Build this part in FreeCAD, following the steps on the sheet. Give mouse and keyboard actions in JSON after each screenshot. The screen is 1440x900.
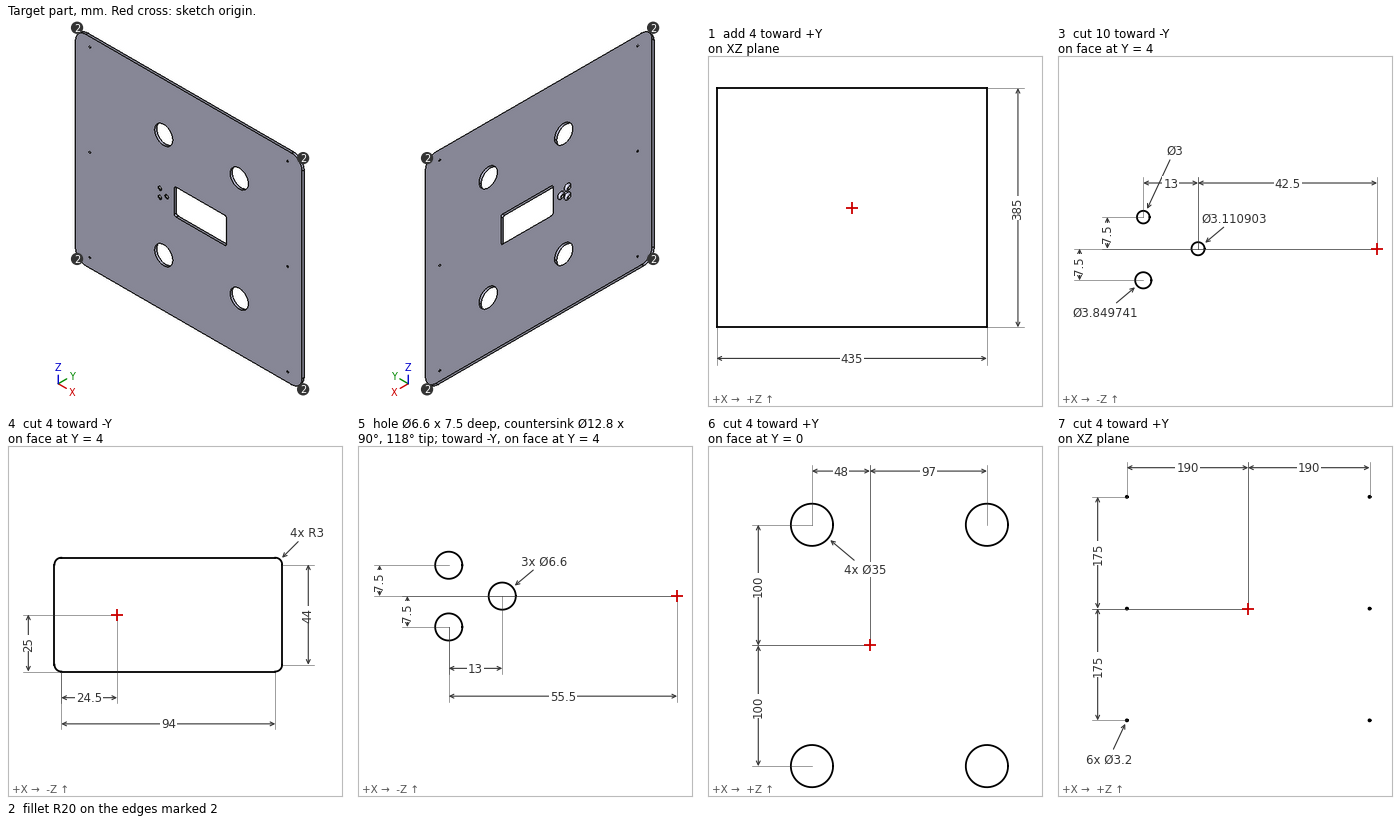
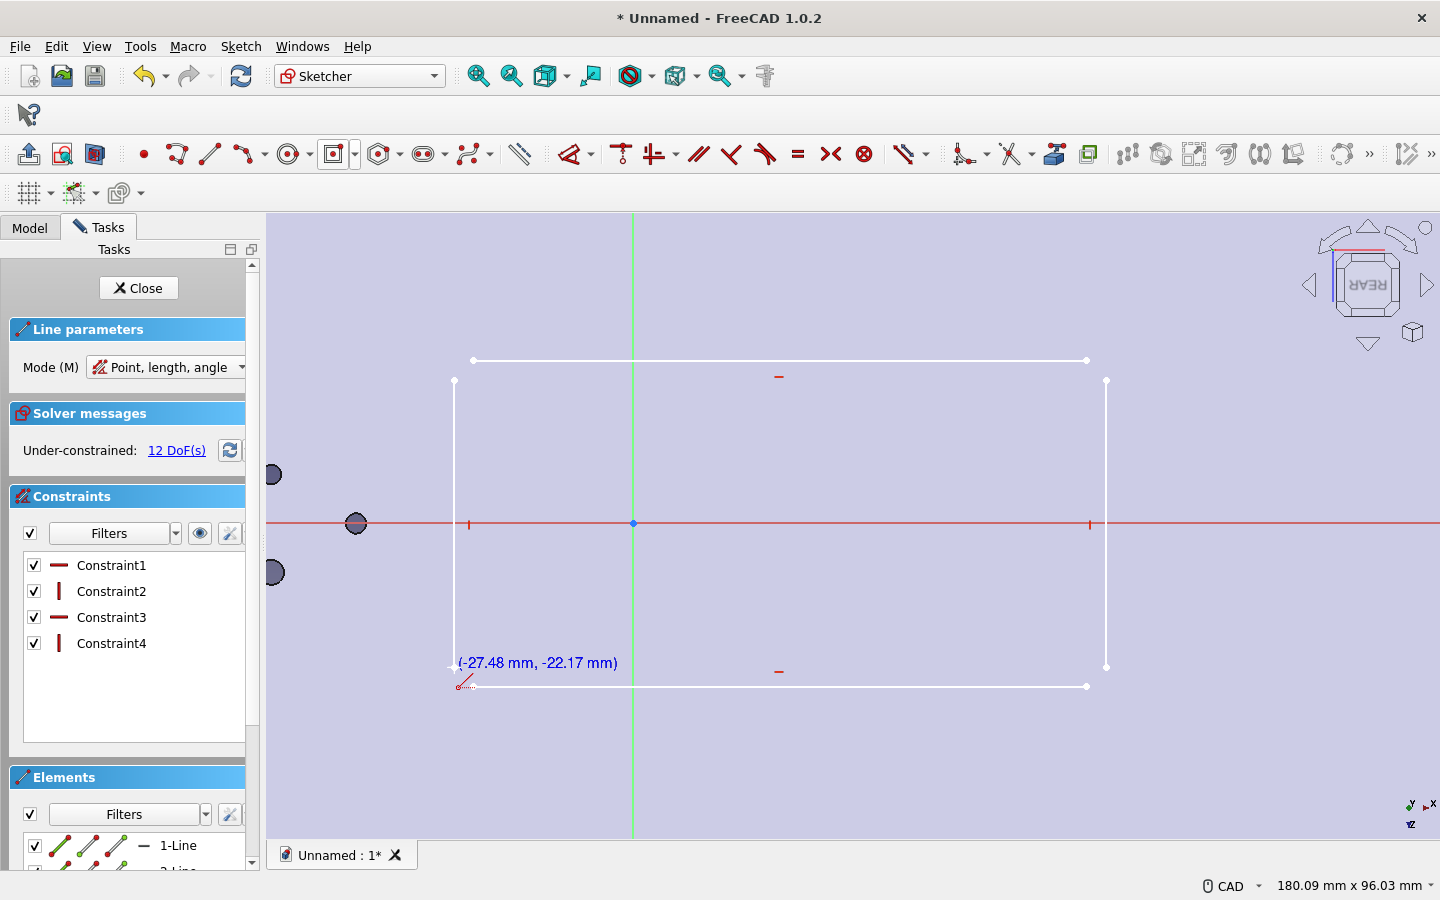
{"action": "left_click", "coordinate": [242, 154]}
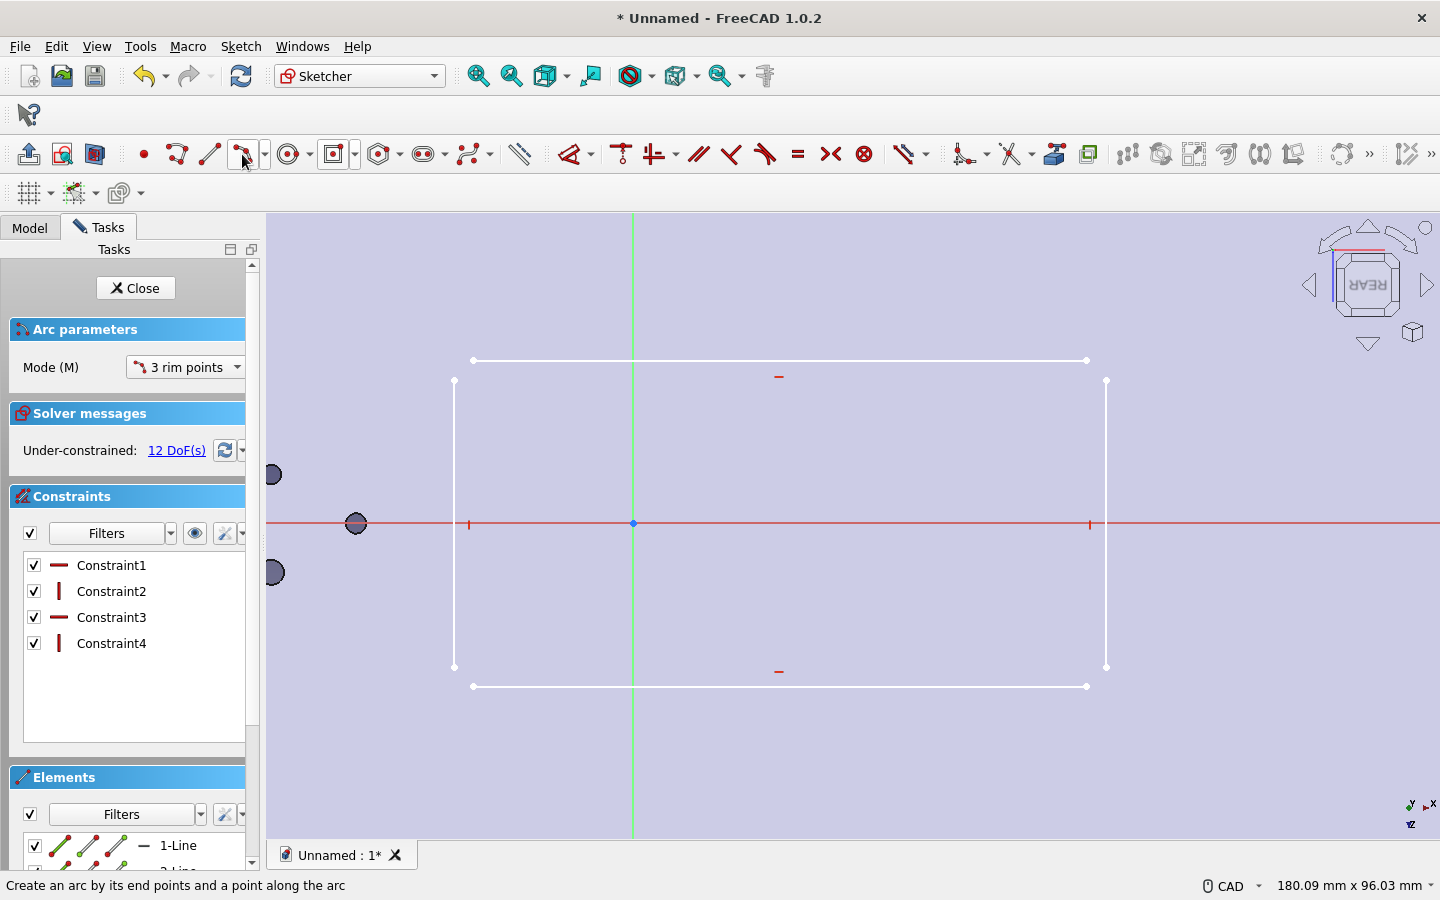
{"action": "left_click", "coordinate": [1086, 687]}
{"action": "left_click", "coordinate": [1106, 668]}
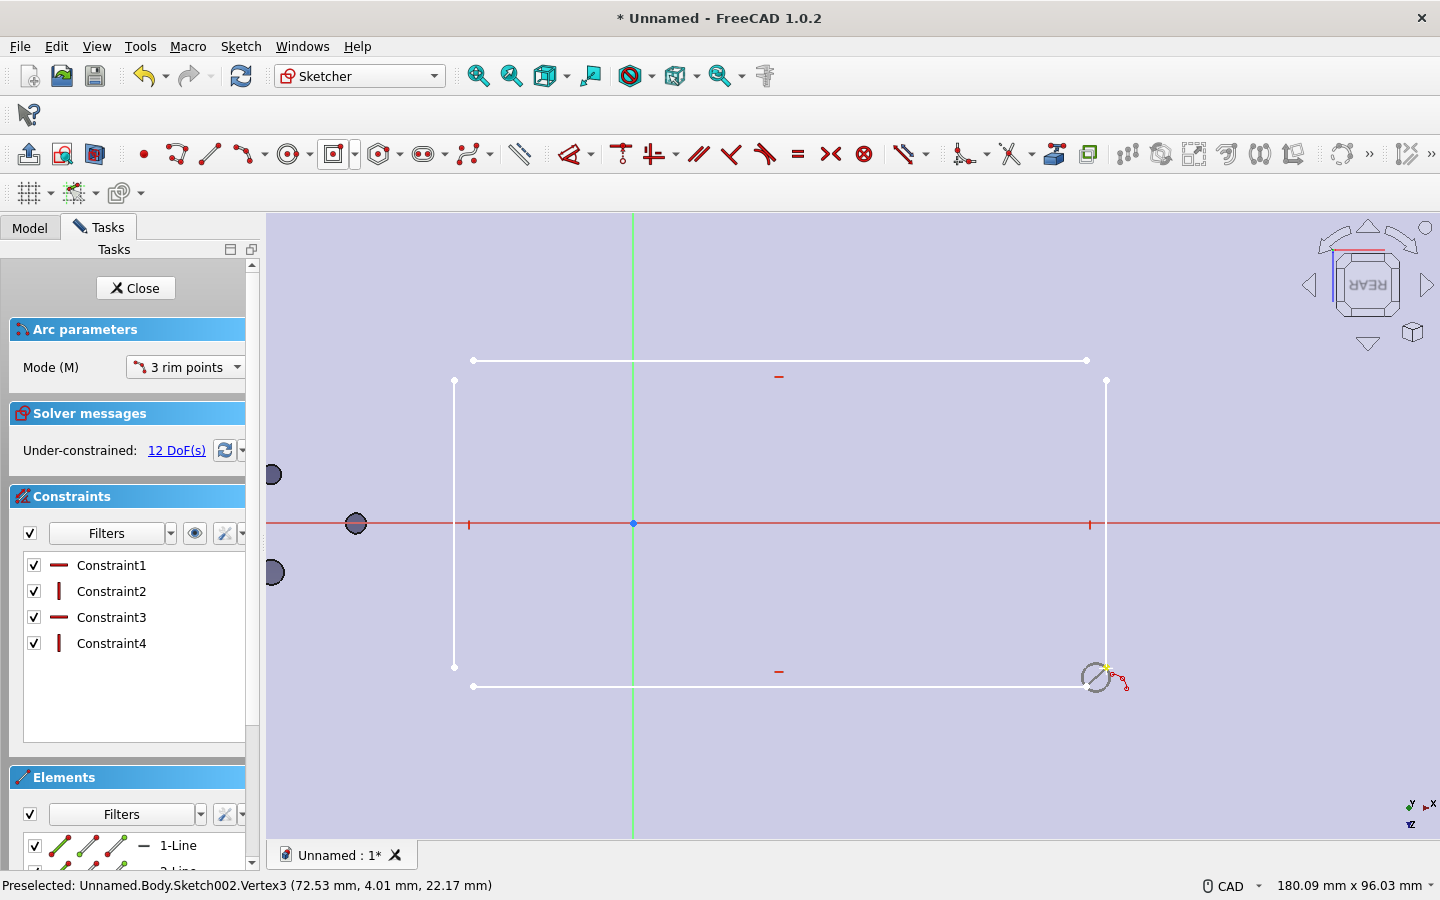
{"action": "scroll", "coordinate": [1100, 681], "scroll_direction": "up", "scroll_amount": 6}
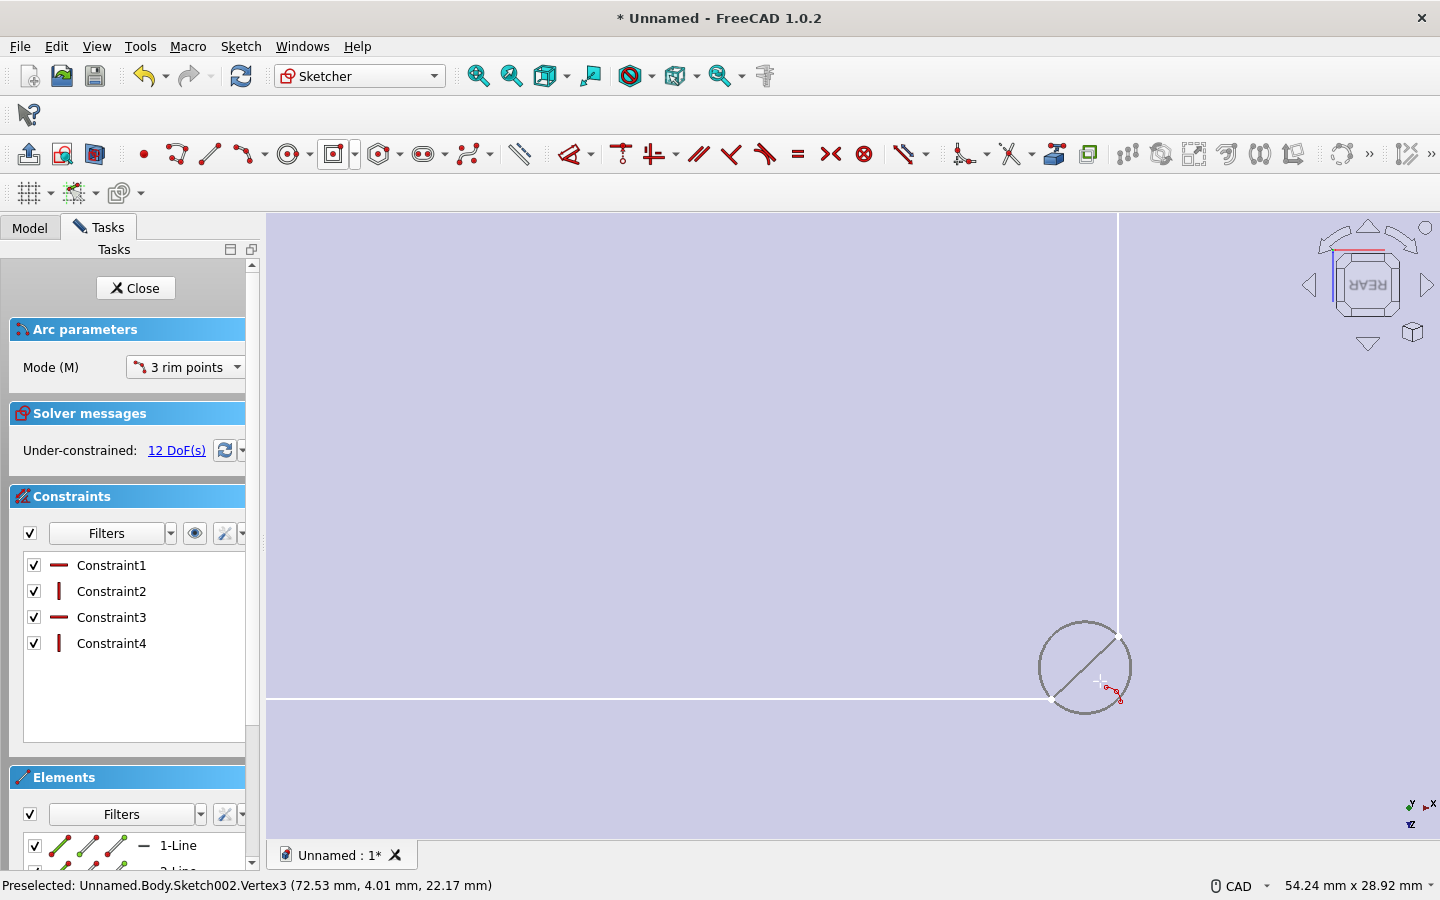
{"action": "left_click", "coordinate": [1099, 678]}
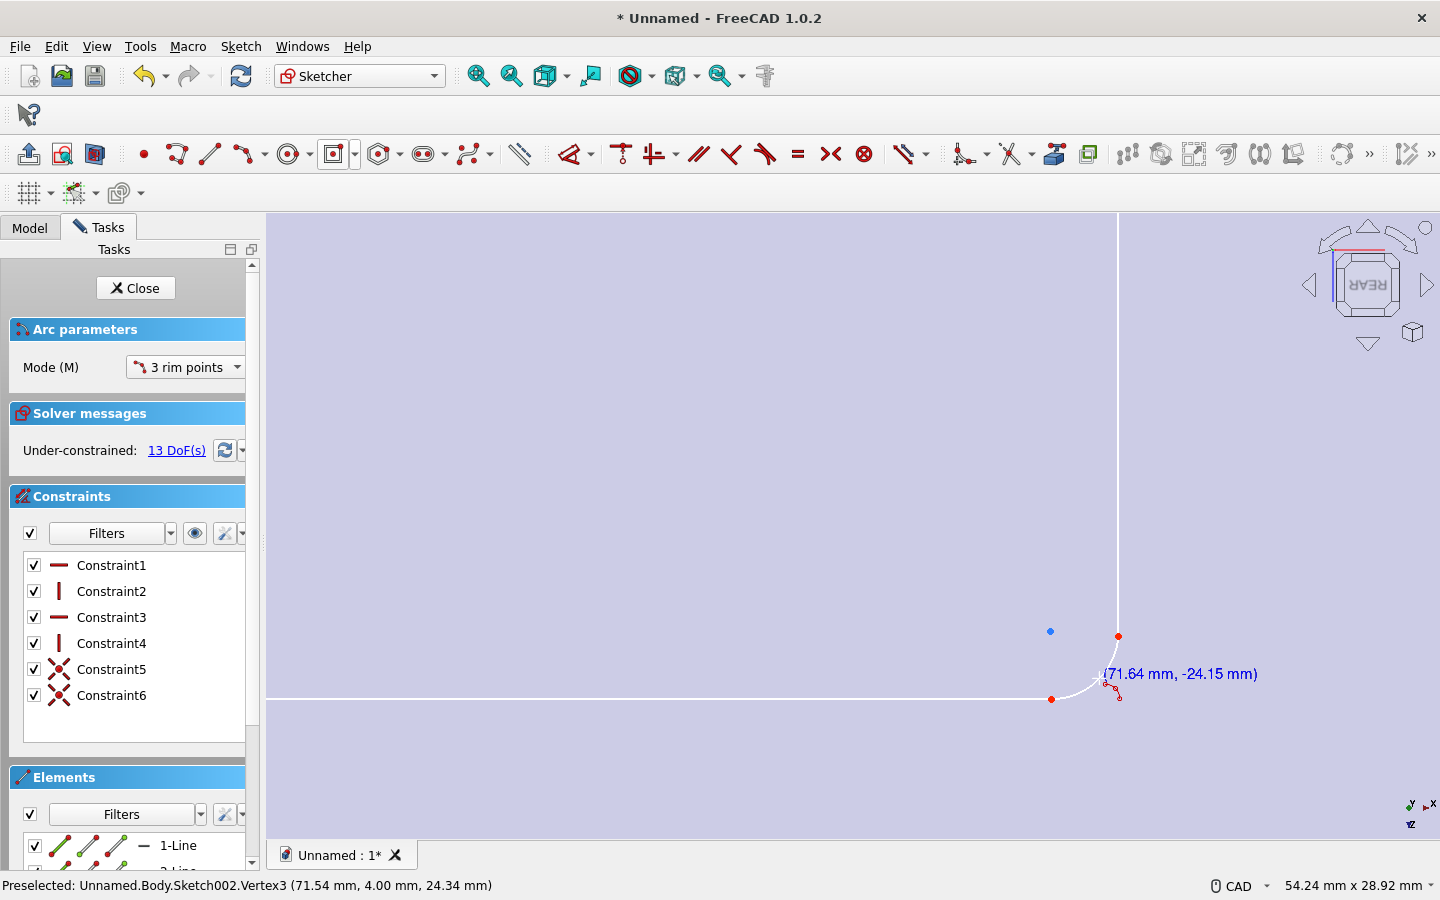
{"action": "scroll", "coordinate": [1107, 685], "scroll_direction": "down", "scroll_amount": 6}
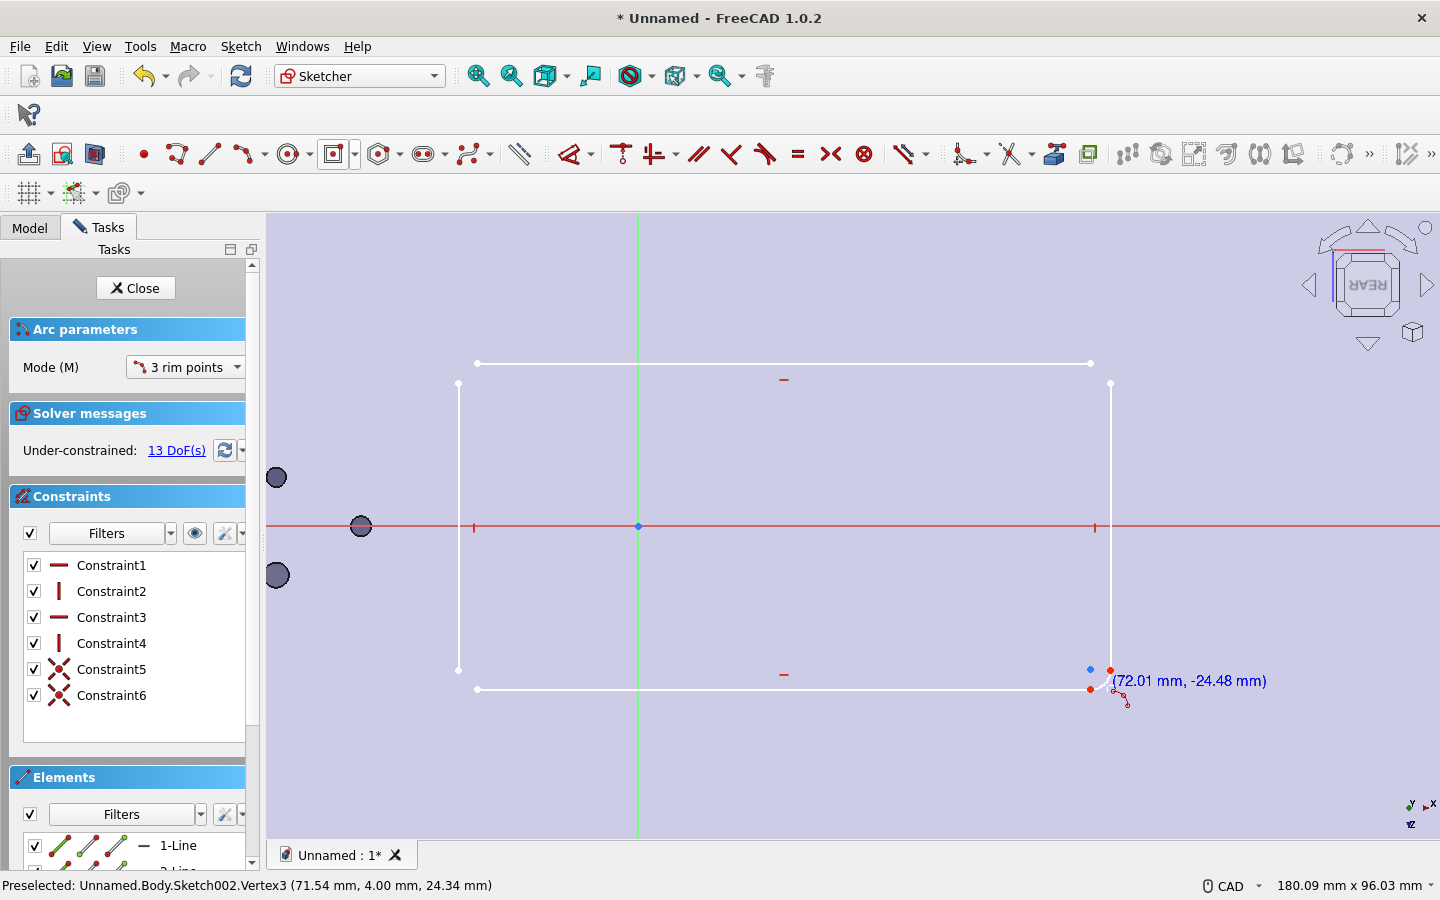
{"action": "left_click", "coordinate": [1111, 384]}
{"action": "left_click", "coordinate": [1091, 364]}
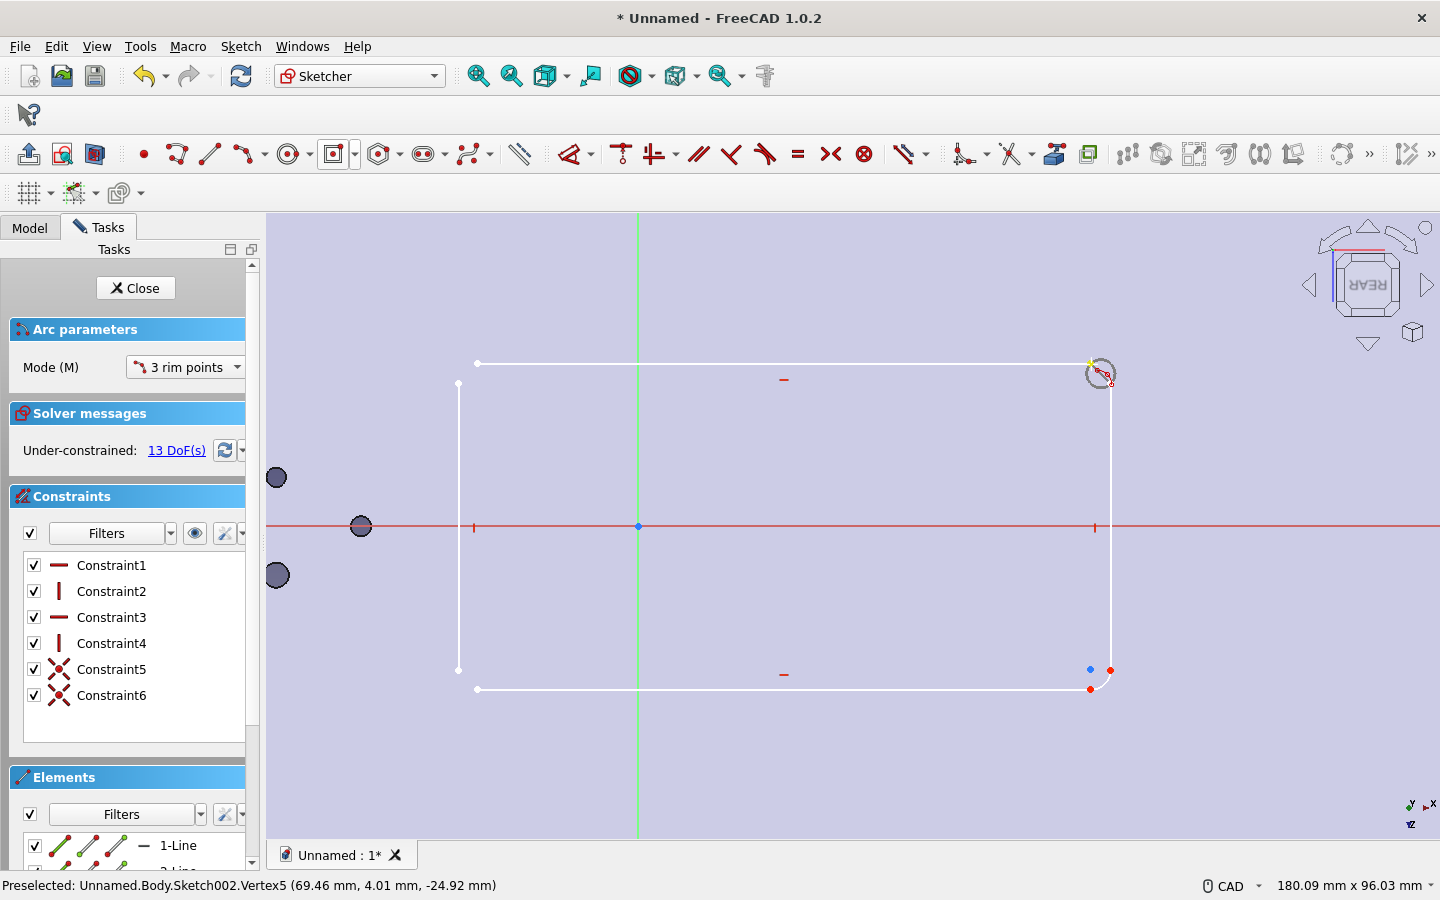
{"action": "scroll", "coordinate": [1105, 369], "scroll_direction": "up", "scroll_amount": 6}